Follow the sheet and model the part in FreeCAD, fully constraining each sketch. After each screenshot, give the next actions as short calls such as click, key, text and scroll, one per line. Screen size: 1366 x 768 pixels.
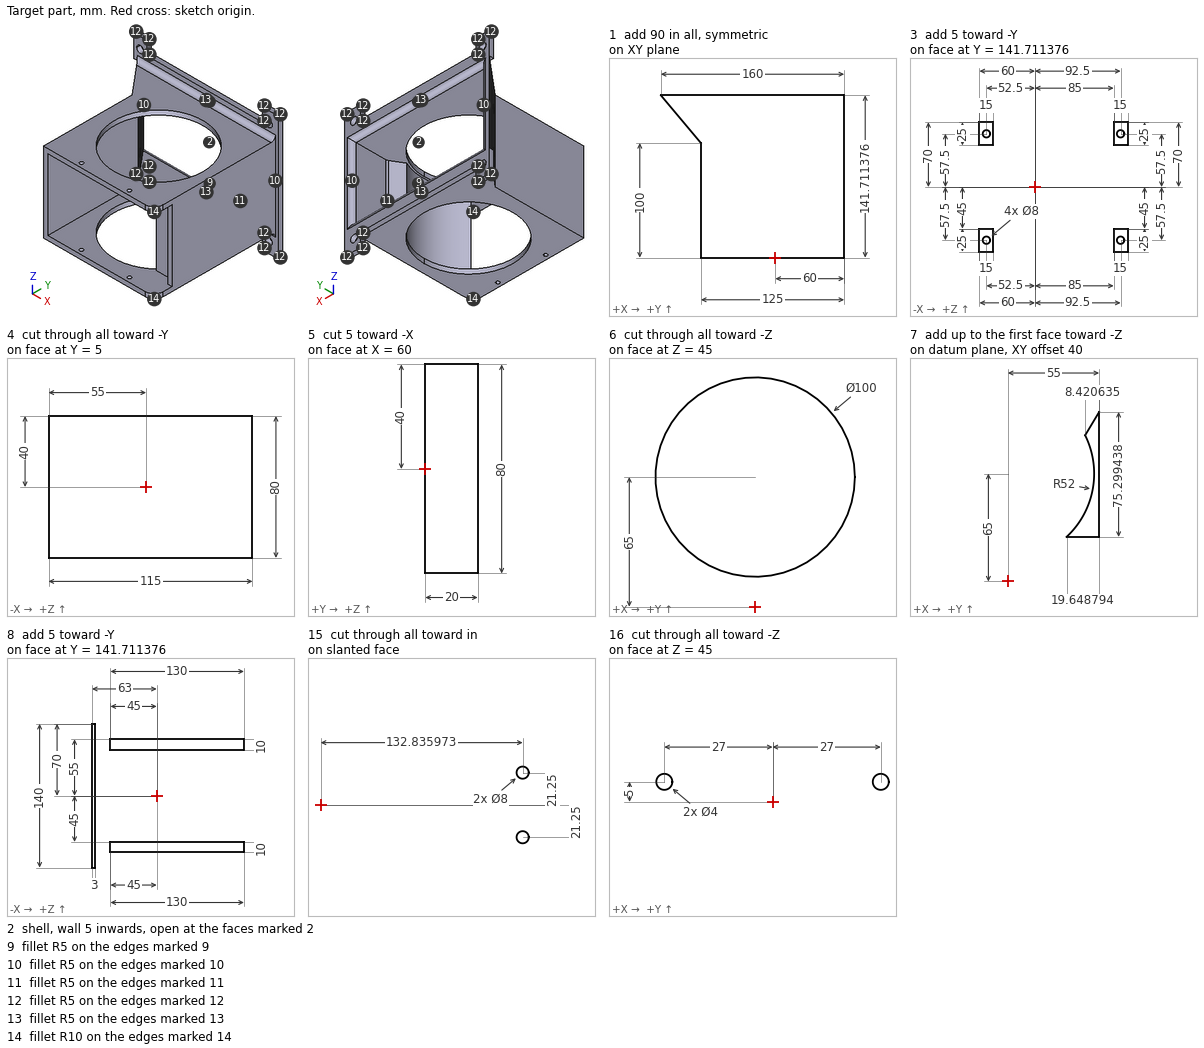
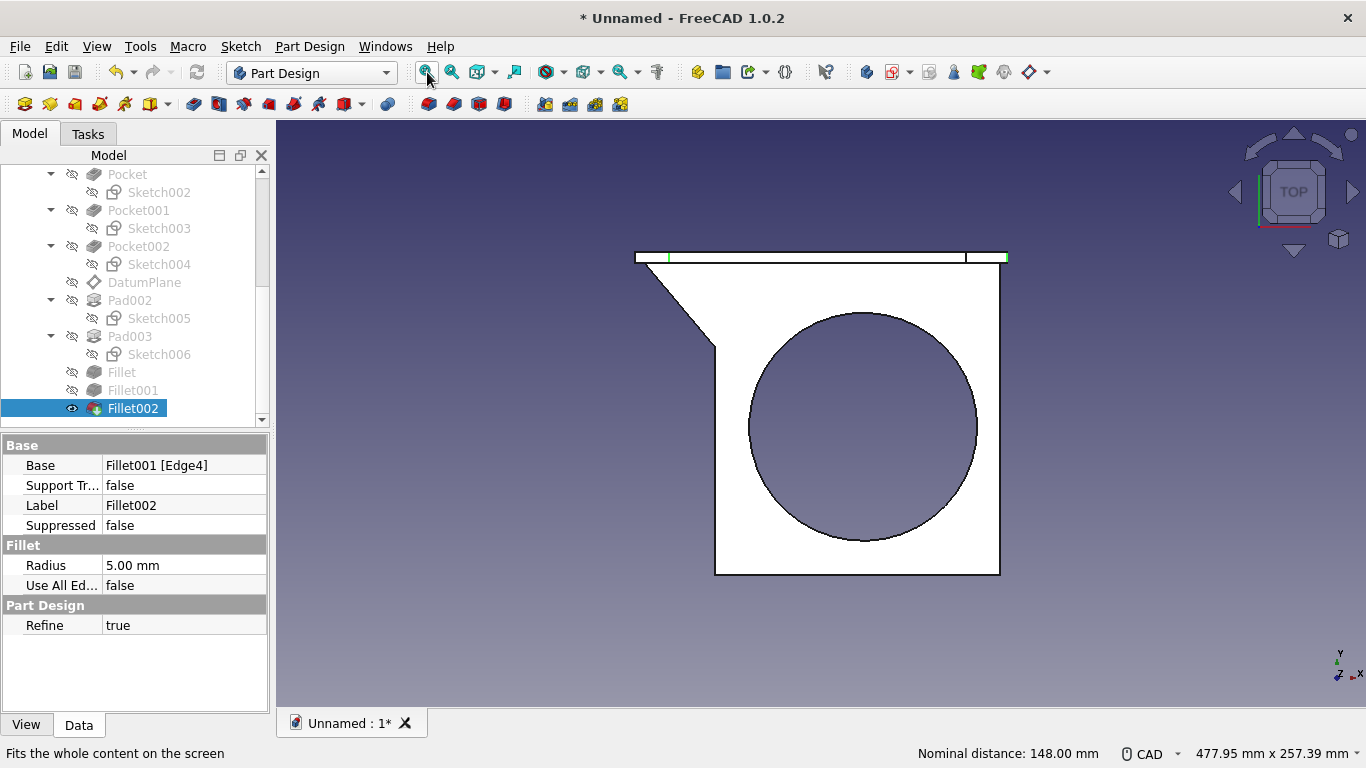
scroll(966, 257, up, 7)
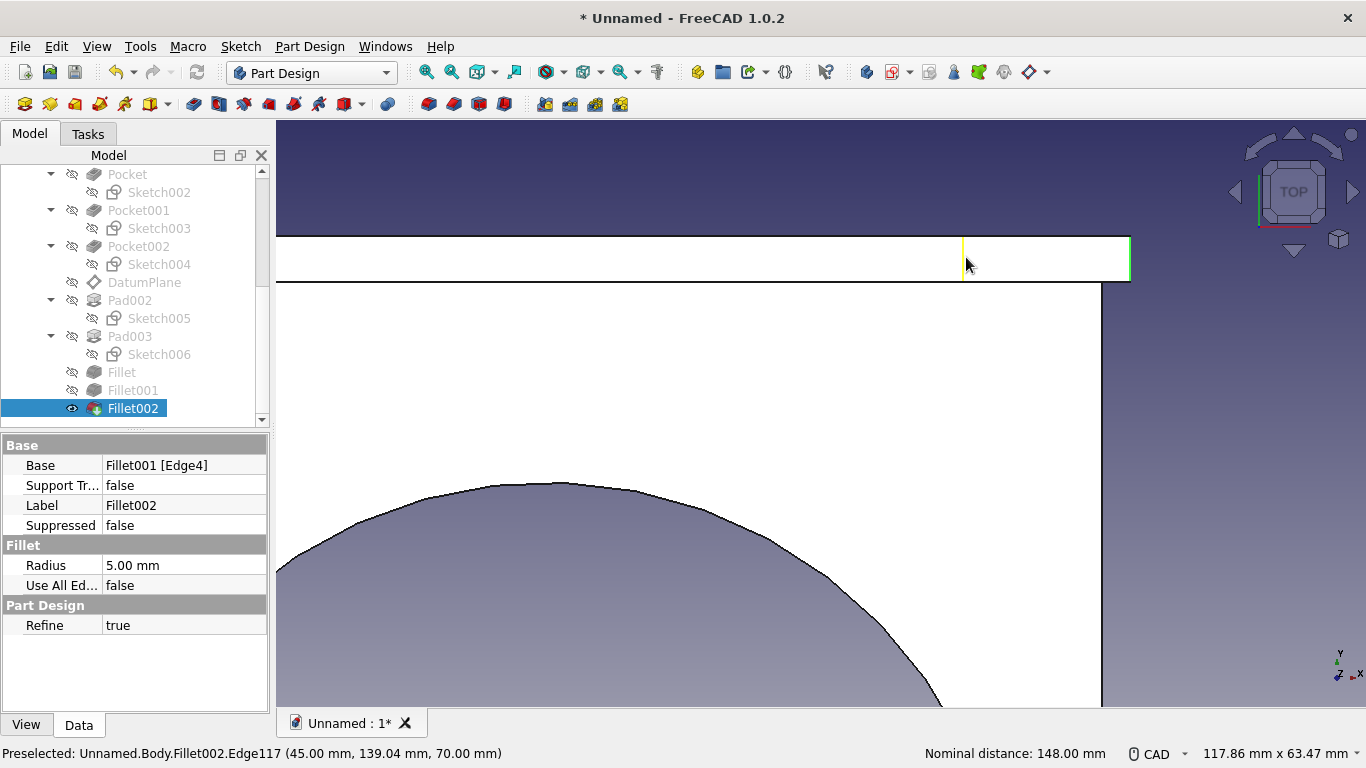
click(963, 258, ctrl)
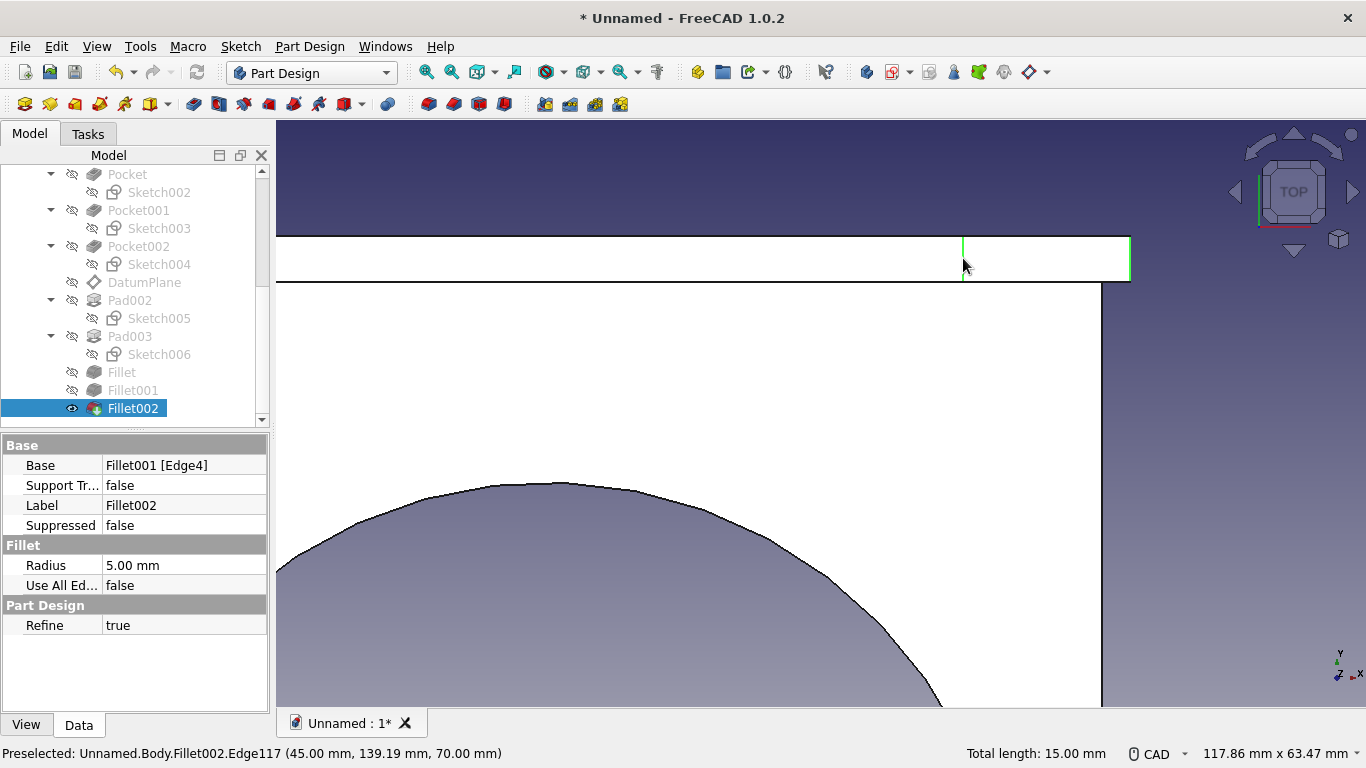
key(v)
key(f)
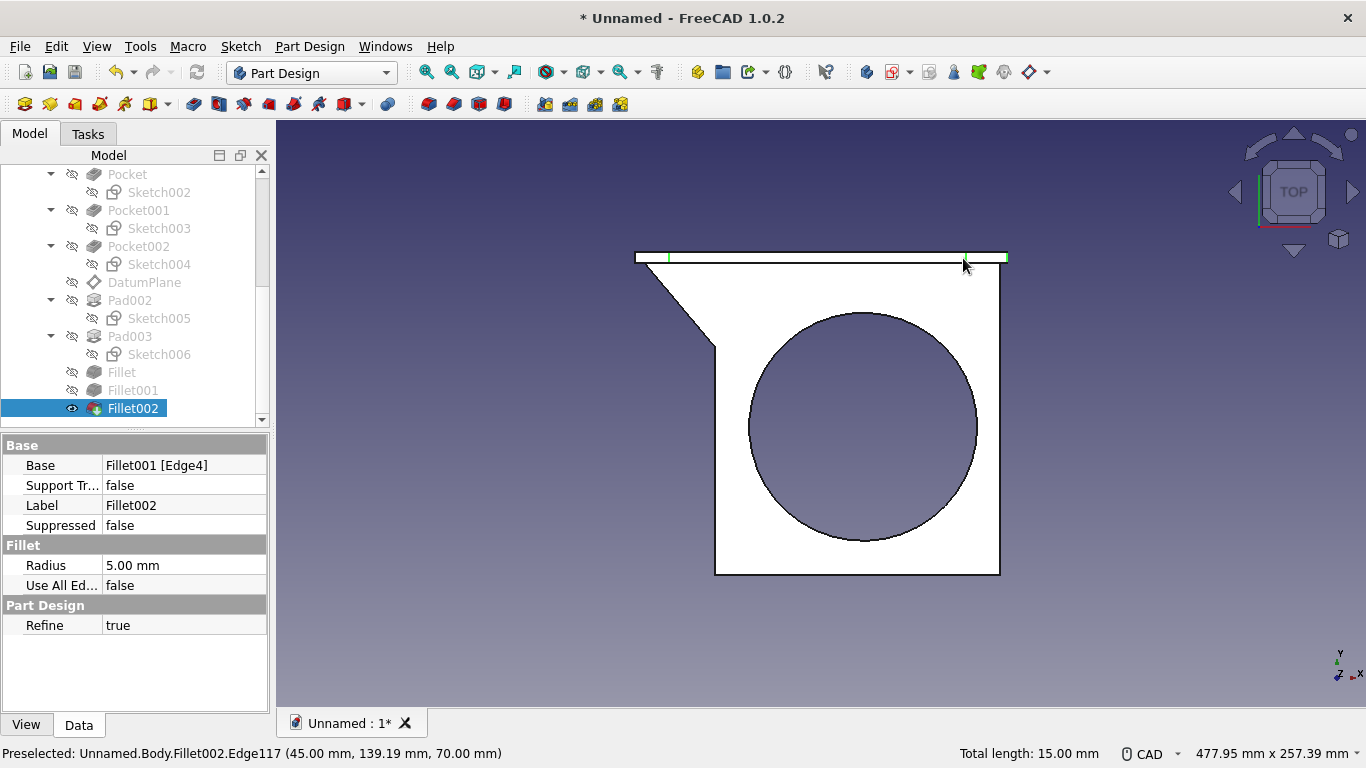
key(0)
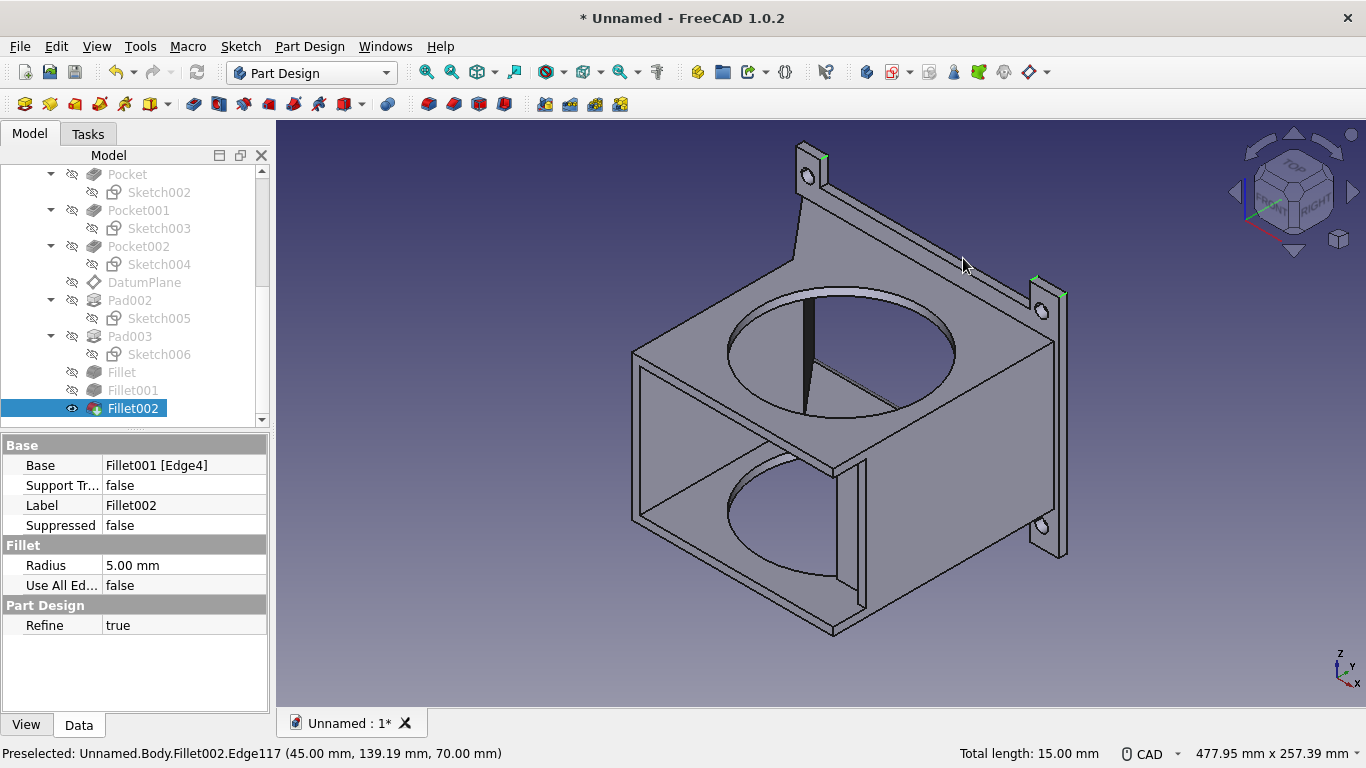
scroll(1034, 510, up, 7)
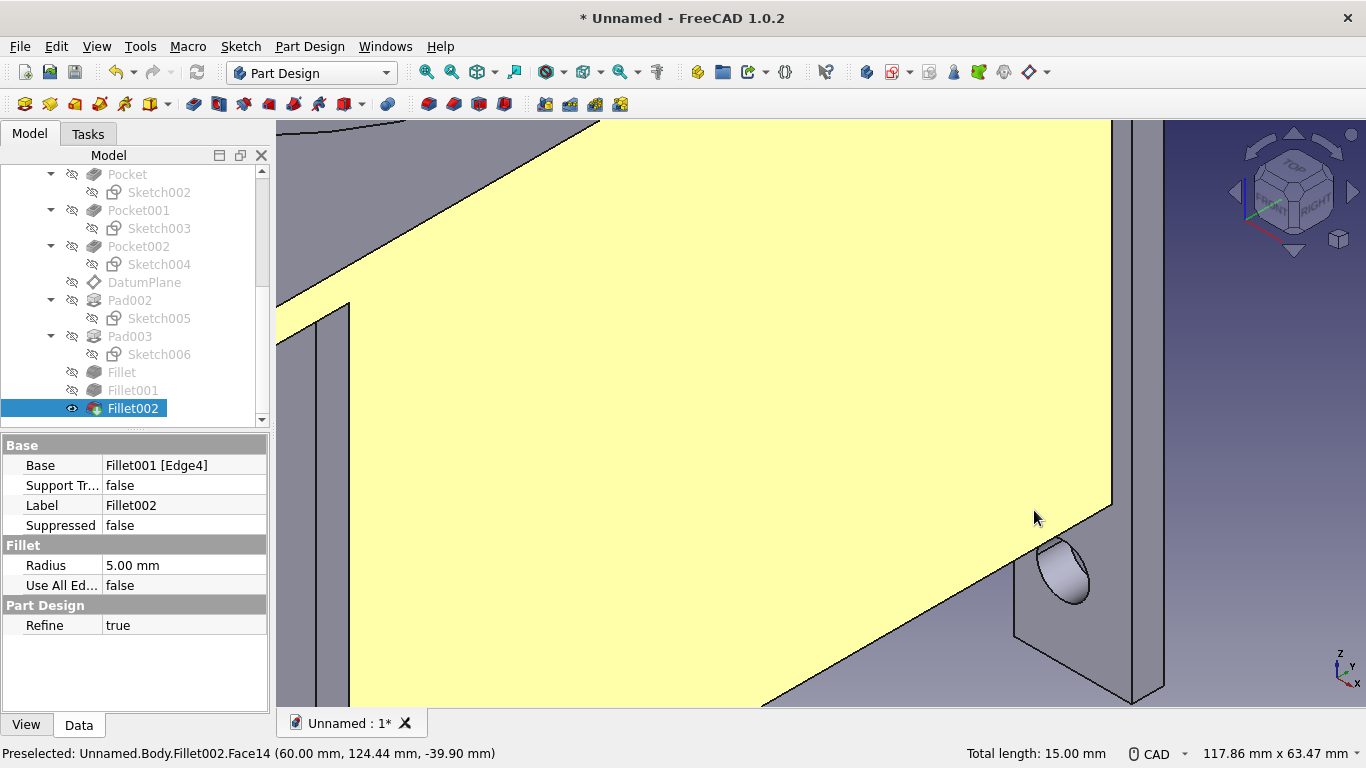
key(v)
key(f)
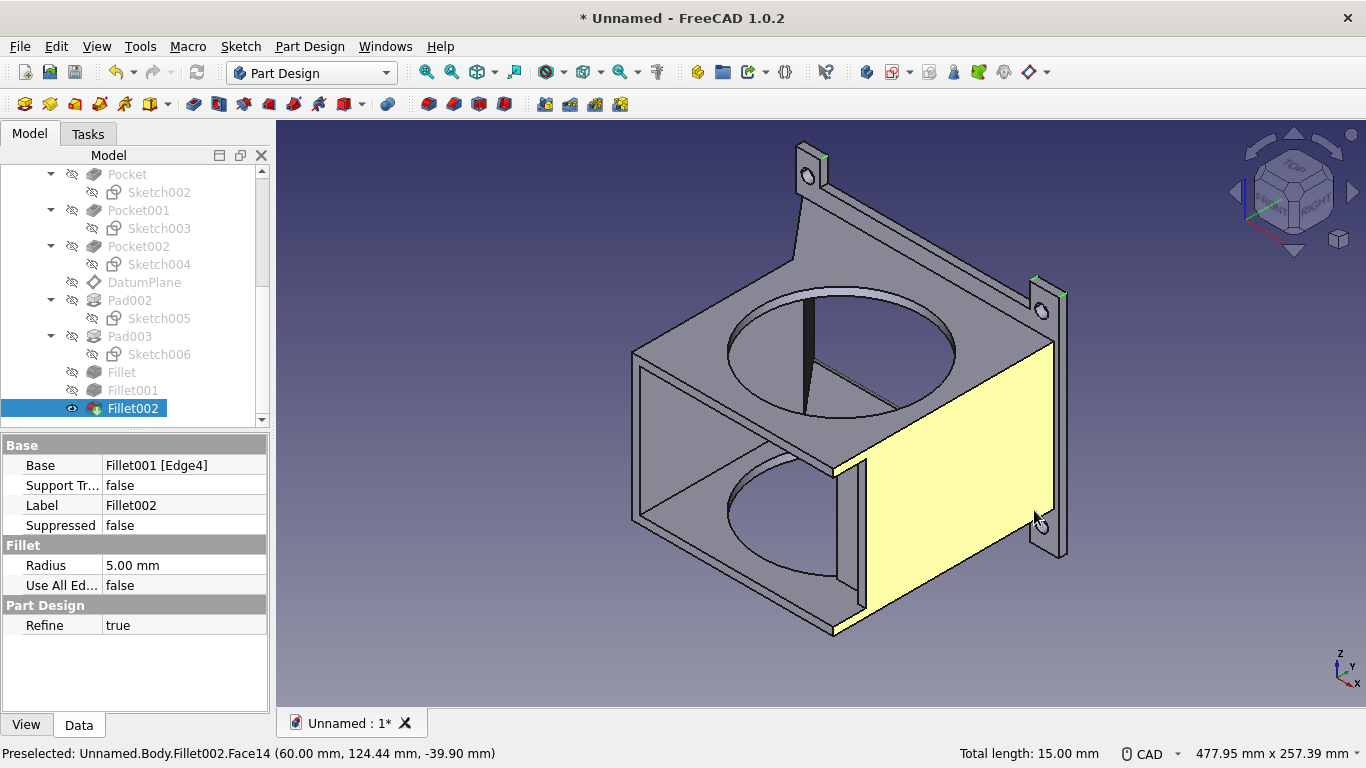
key(1)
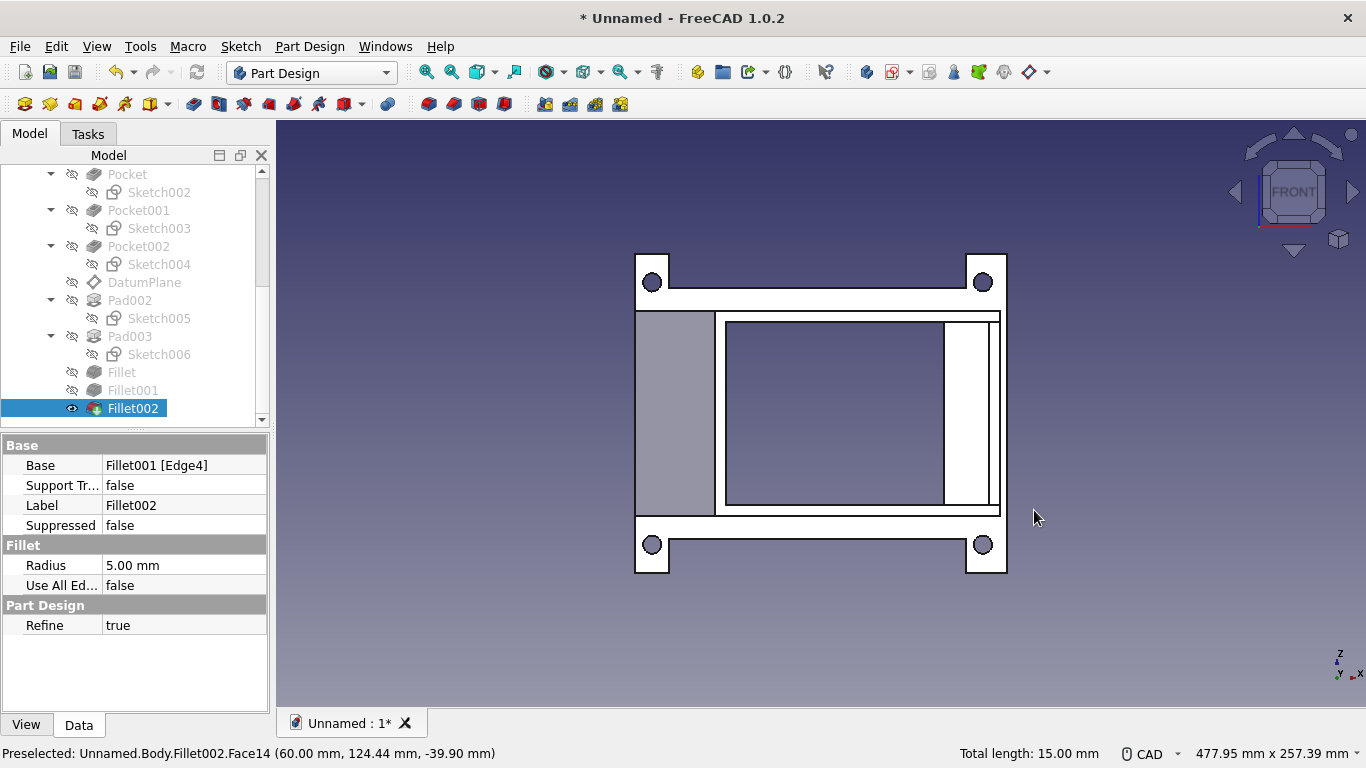
scroll(966, 538, up, 7)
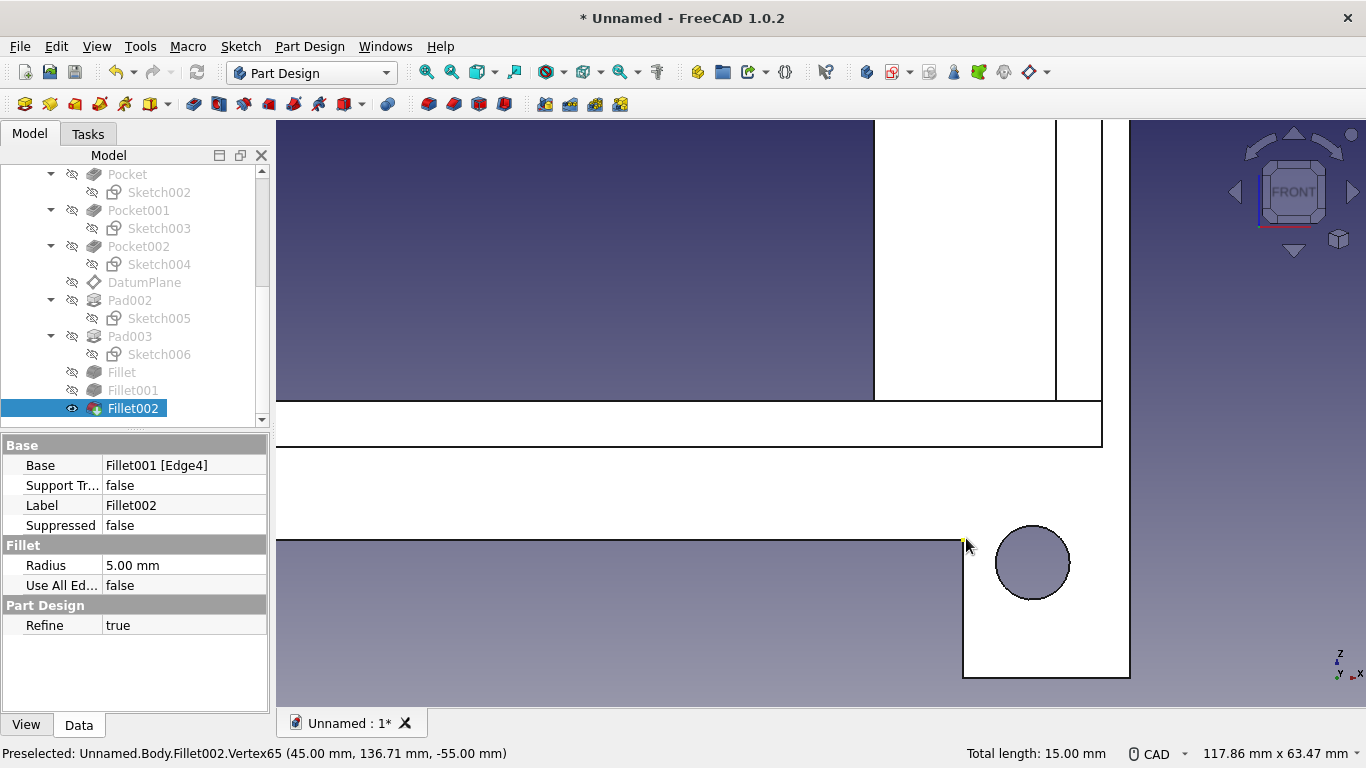
key(v)
key(f)